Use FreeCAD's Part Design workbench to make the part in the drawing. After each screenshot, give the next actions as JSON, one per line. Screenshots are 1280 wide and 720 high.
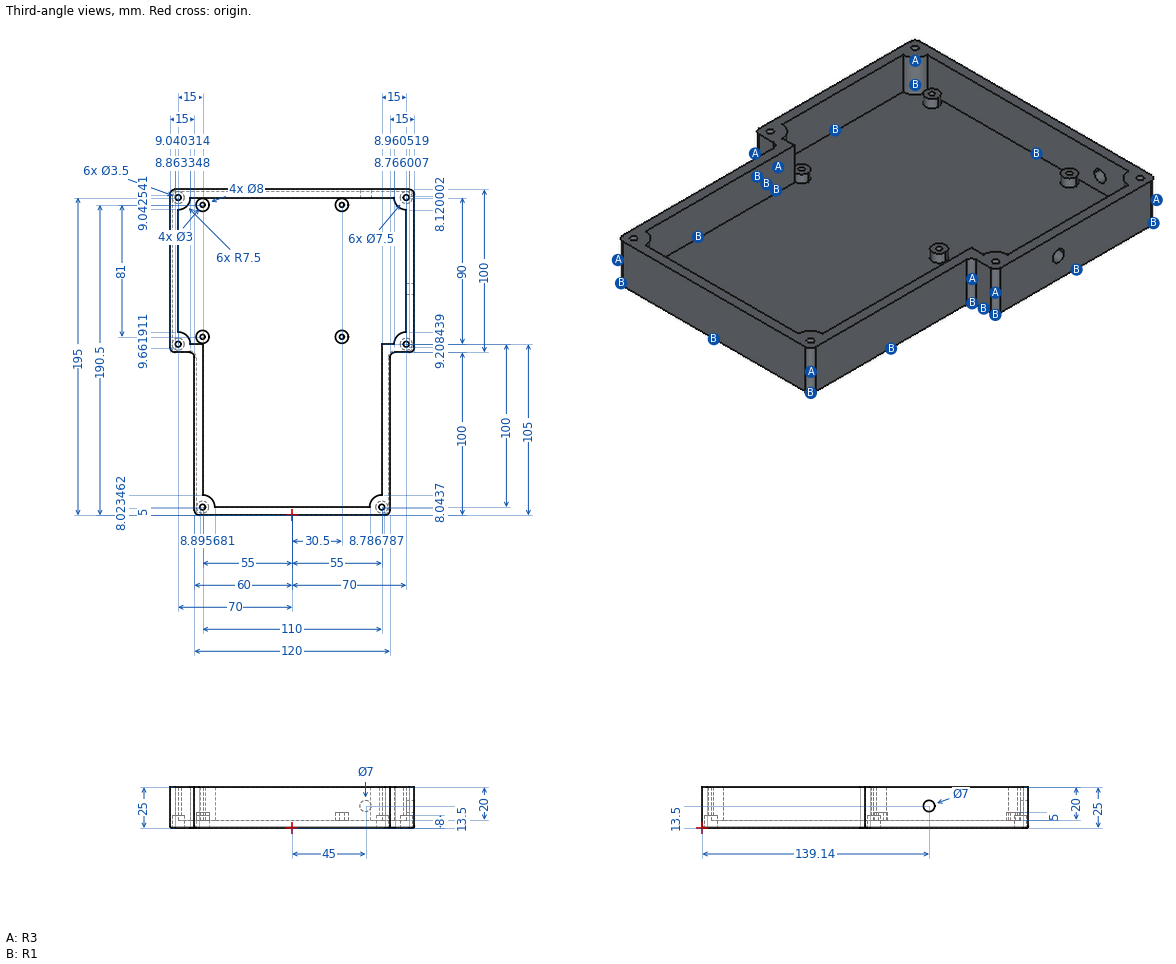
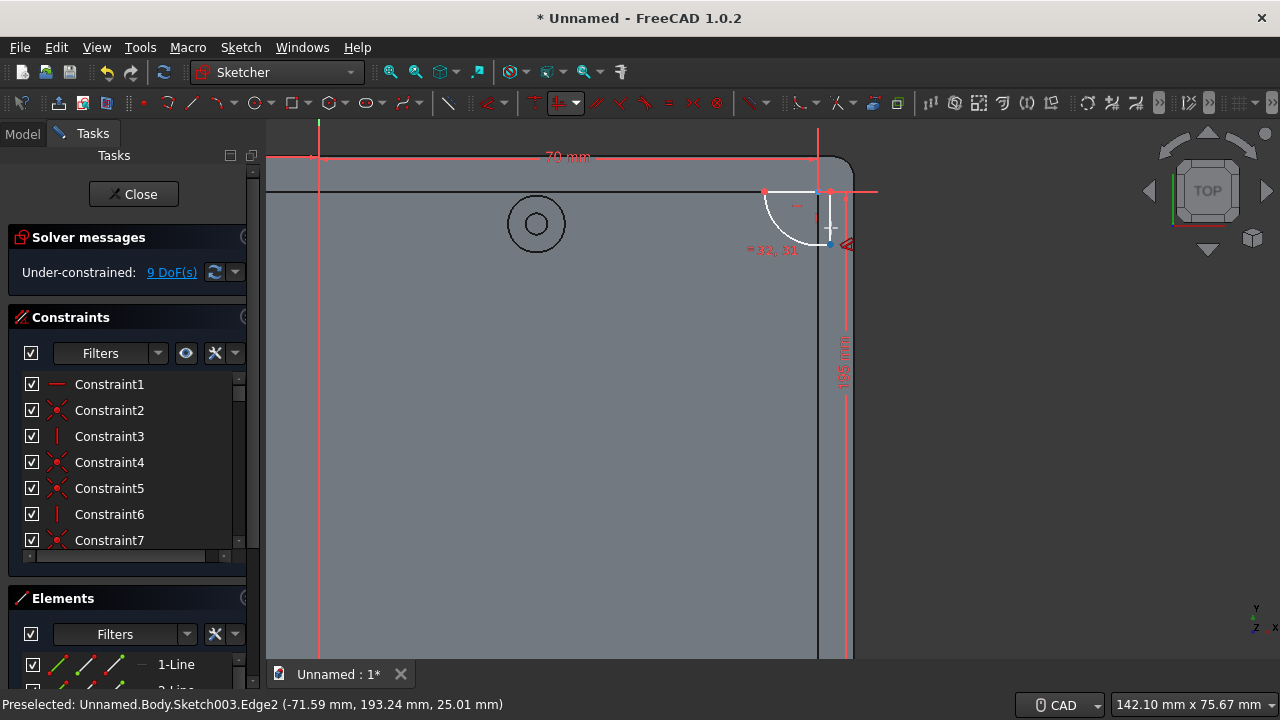
{"action": "left_click", "coordinate": [830, 228]}
{"action": "left_click", "coordinate": [864, 218]}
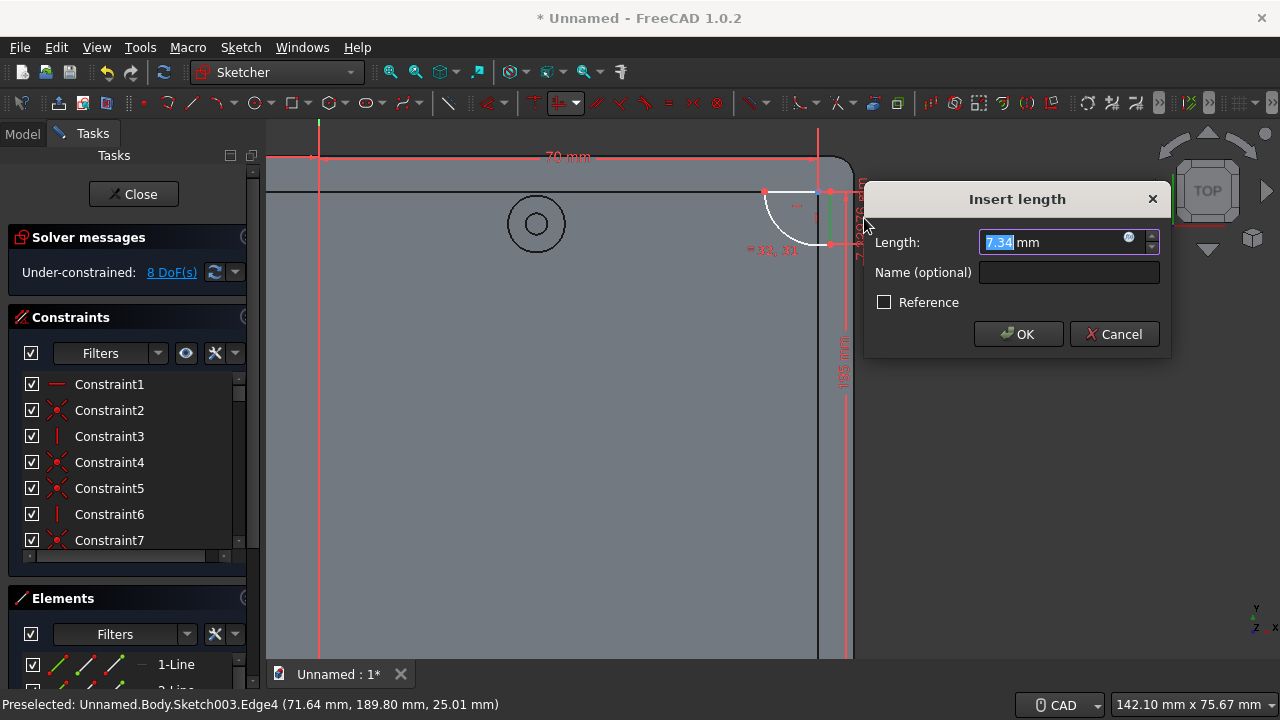
{"action": "type", "text": "8.120002"}
{"action": "key", "text": "Return"}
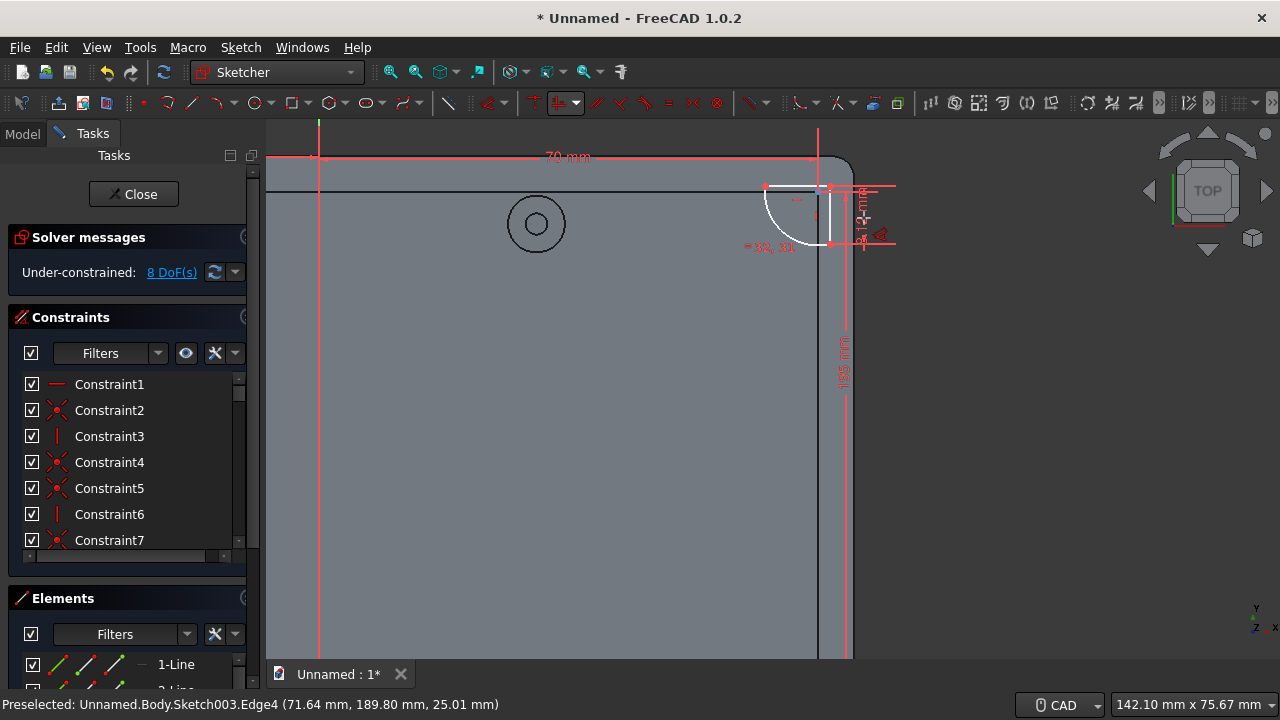
{"action": "left_click", "coordinate": [811, 186]}
{"action": "left_click", "coordinate": [798, 152]}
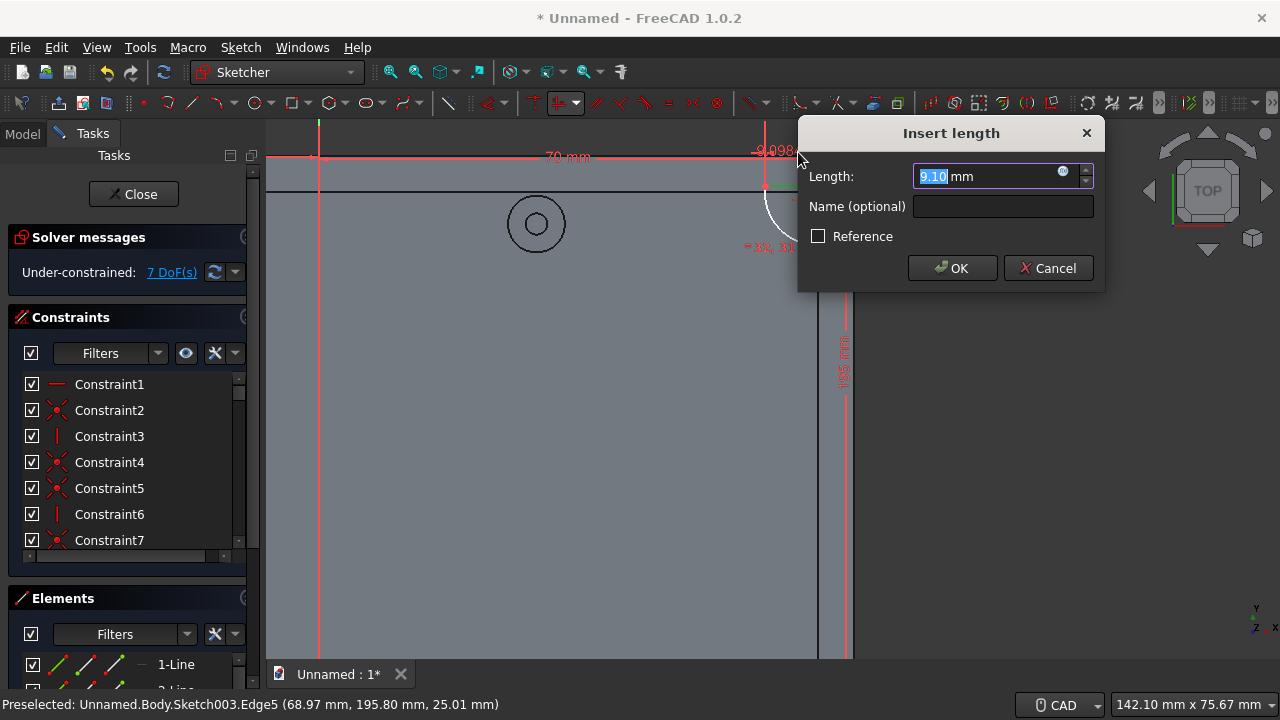
{"action": "type", "text": "8.960519"}
{"action": "key", "text": "Return"}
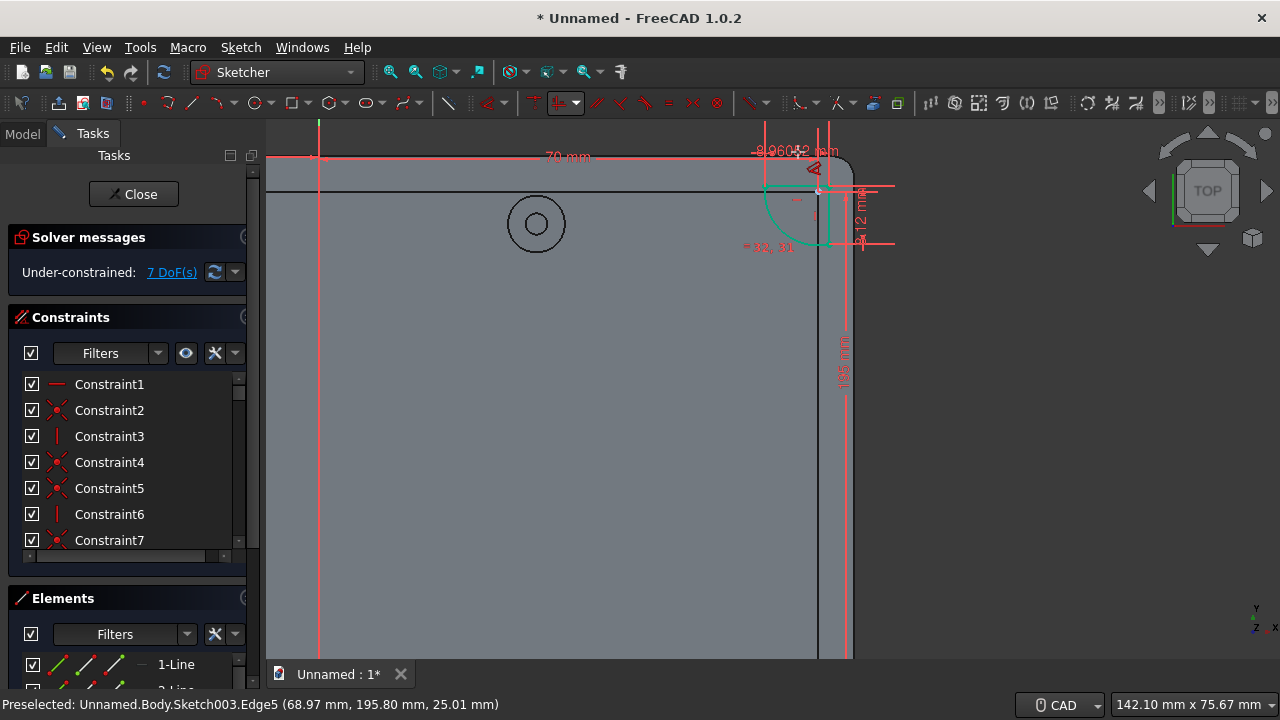
{"action": "scroll", "coordinate": [831, 228], "scroll_direction": "down", "scroll_amount": 7}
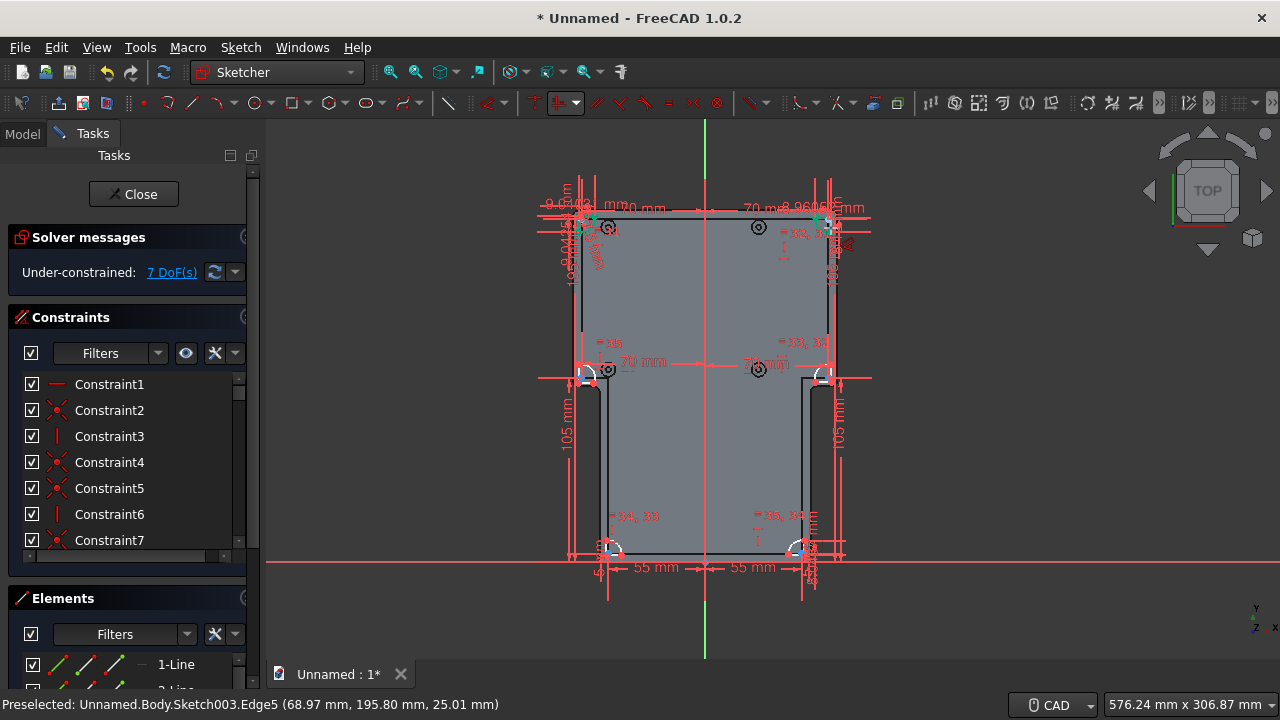
{"action": "scroll", "coordinate": [820, 382], "scroll_direction": "up", "scroll_amount": 6}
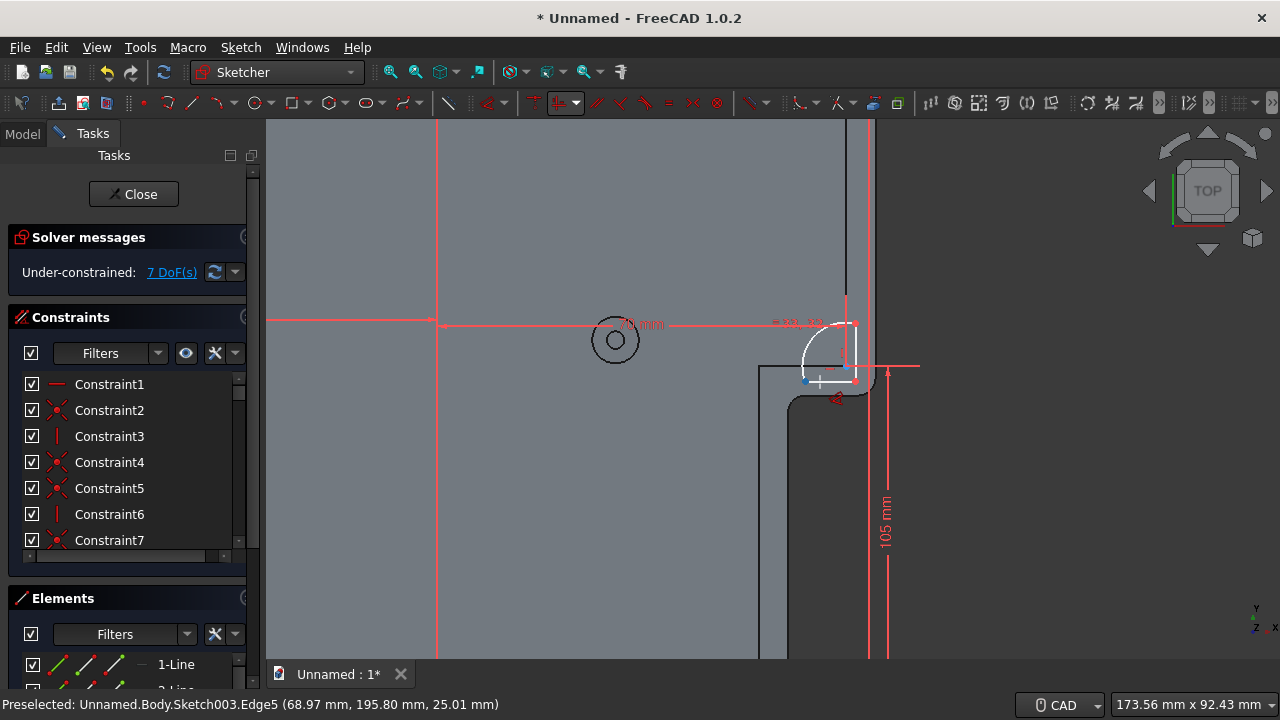
{"action": "left_click", "coordinate": [820, 382]}
{"action": "left_click", "coordinate": [830, 348]}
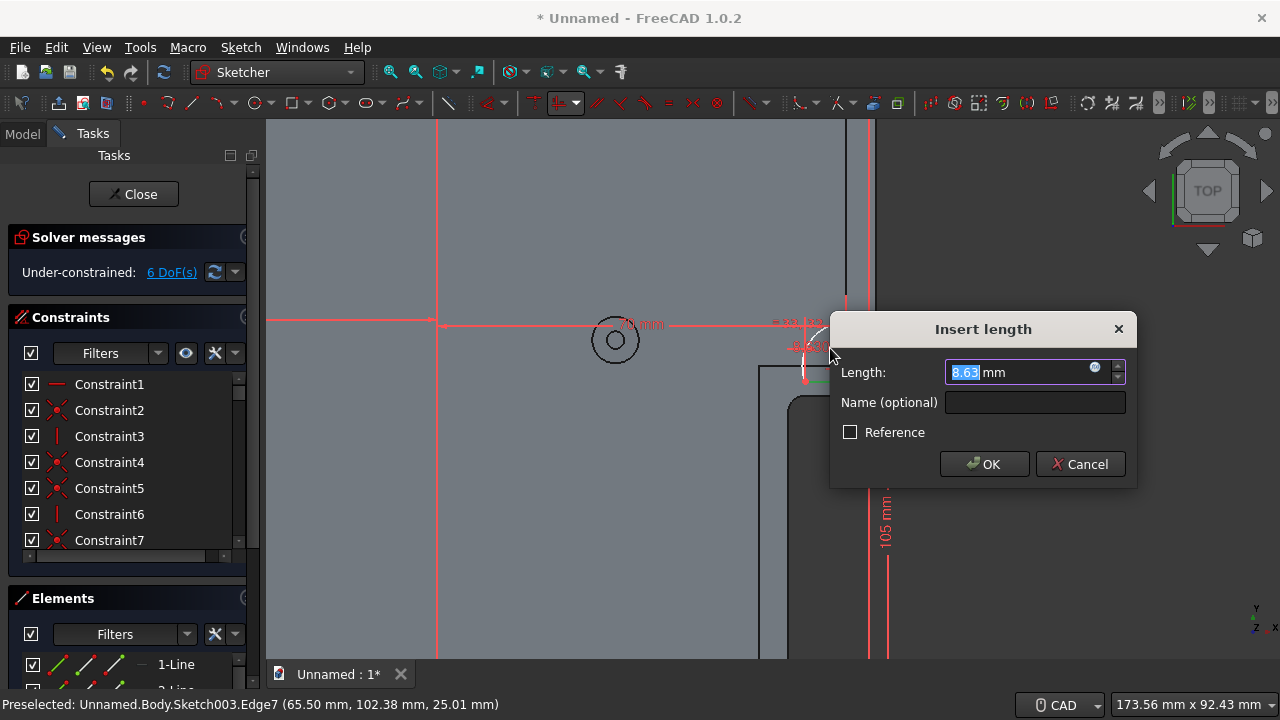
{"action": "type", "text": "8.766007"}
{"action": "key", "text": "Return"}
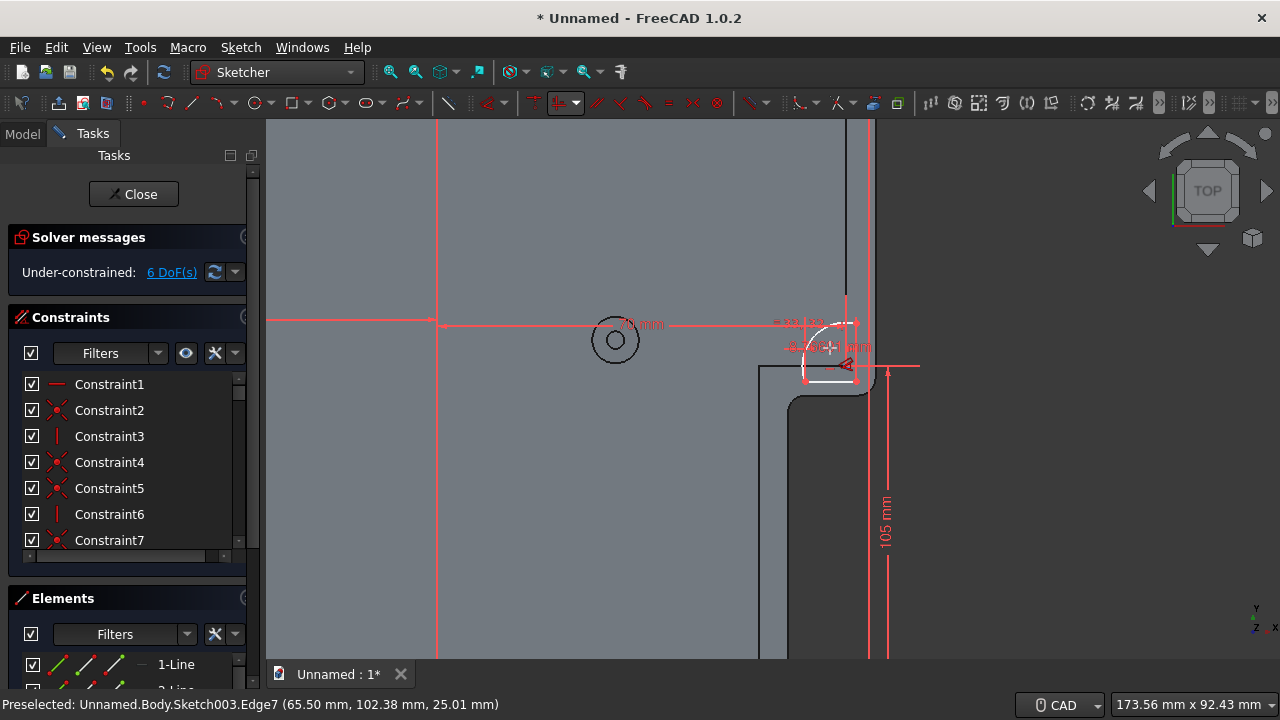
{"action": "left_click", "coordinate": [856, 364]}
{"action": "left_click", "coordinate": [890, 373]}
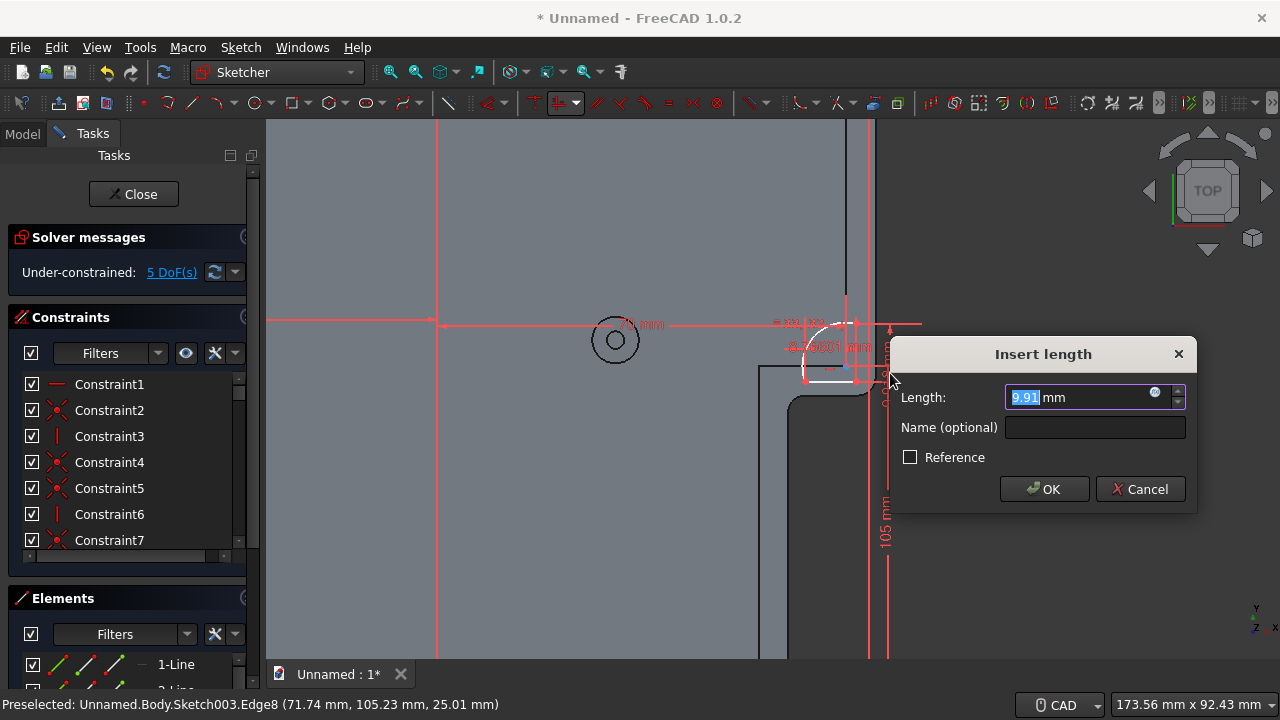
{"action": "type", "text": "9.208439"}
{"action": "key", "text": "Return"}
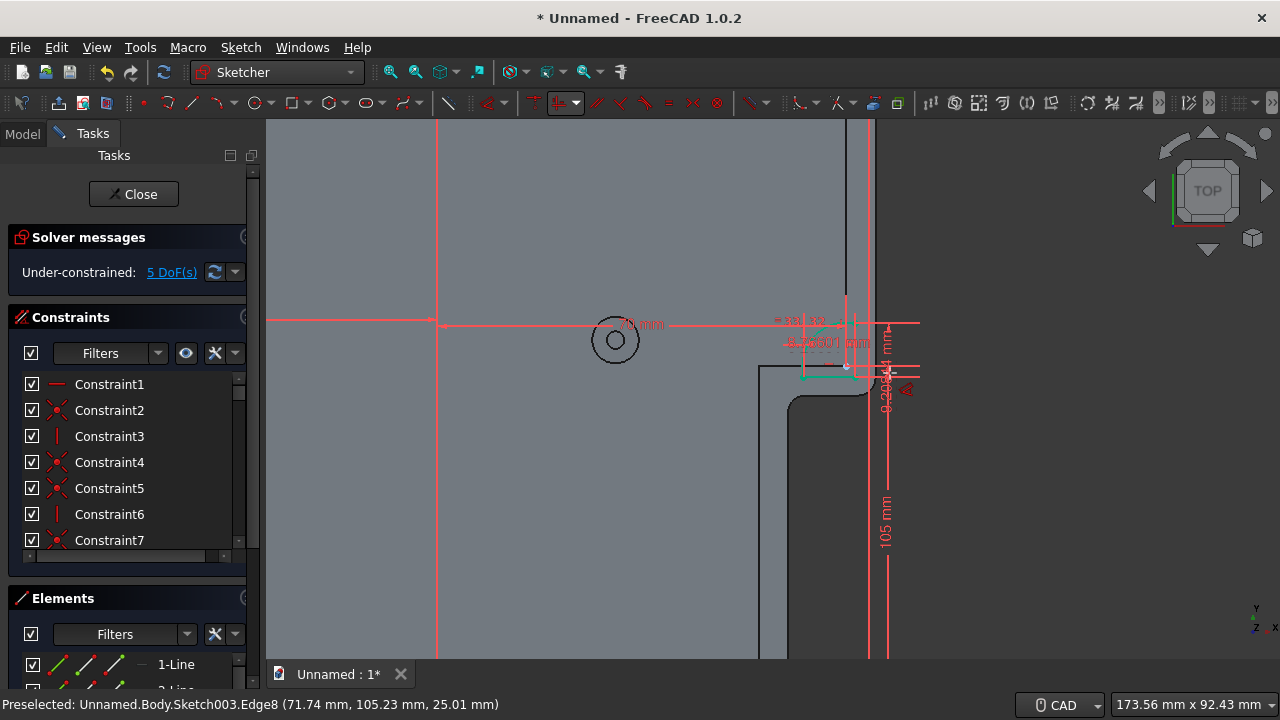
{"action": "scroll", "coordinate": [820, 382], "scroll_direction": "down", "scroll_amount": 6}